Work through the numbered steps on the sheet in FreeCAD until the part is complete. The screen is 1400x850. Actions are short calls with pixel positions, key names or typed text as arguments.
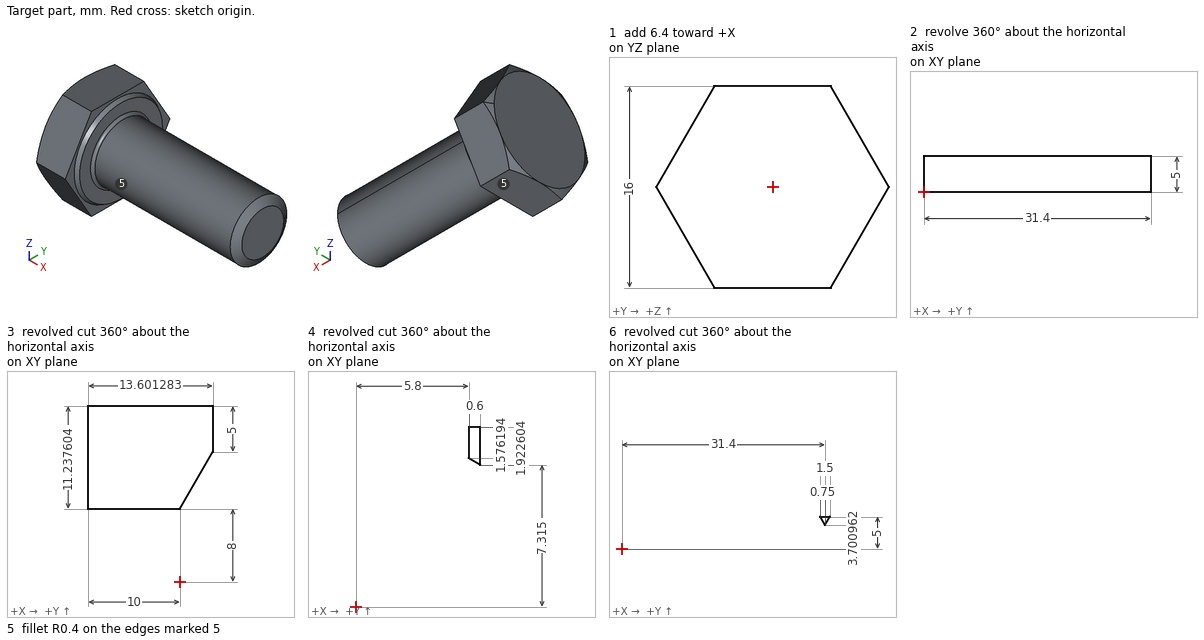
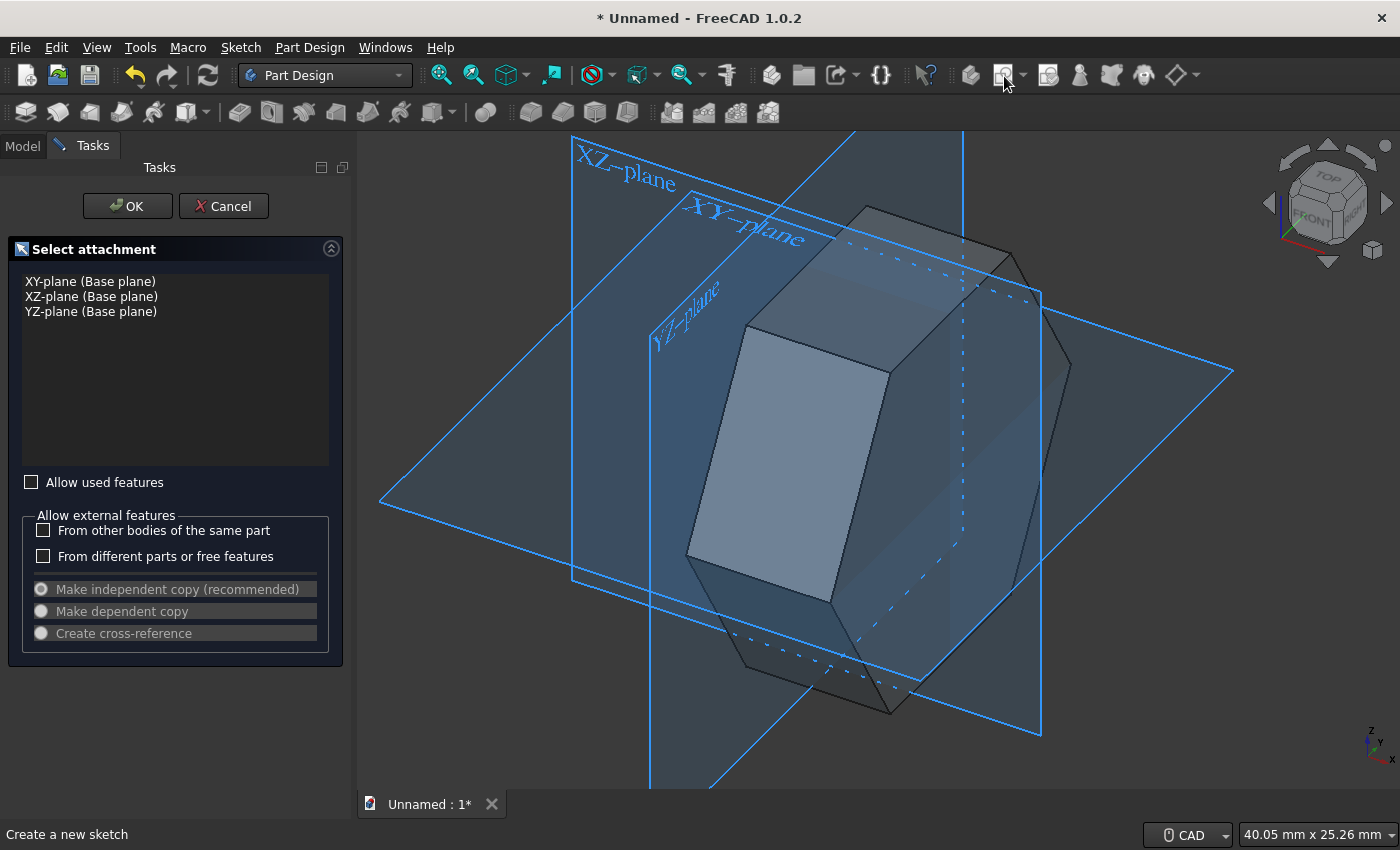
click(82, 282)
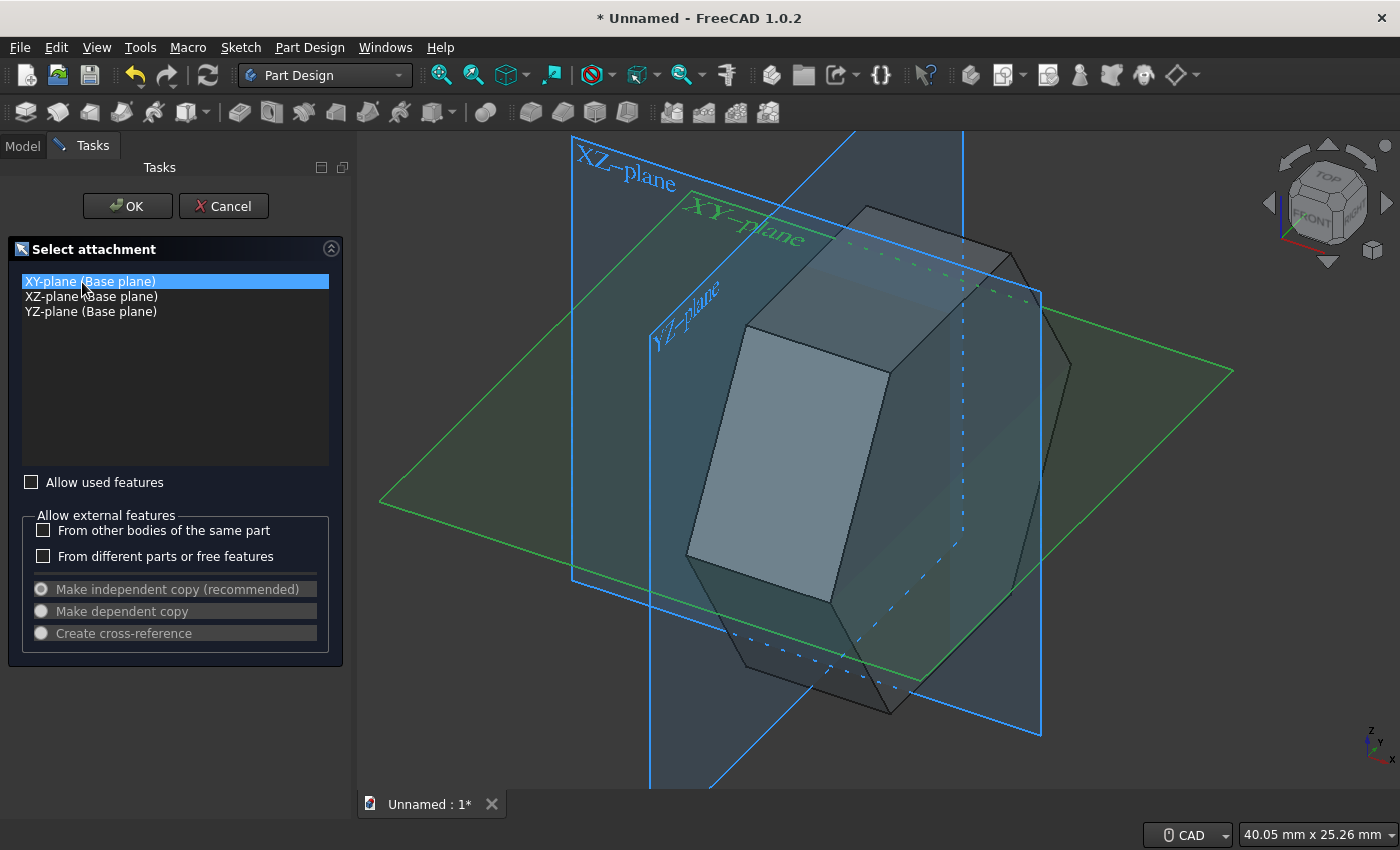
click(128, 206)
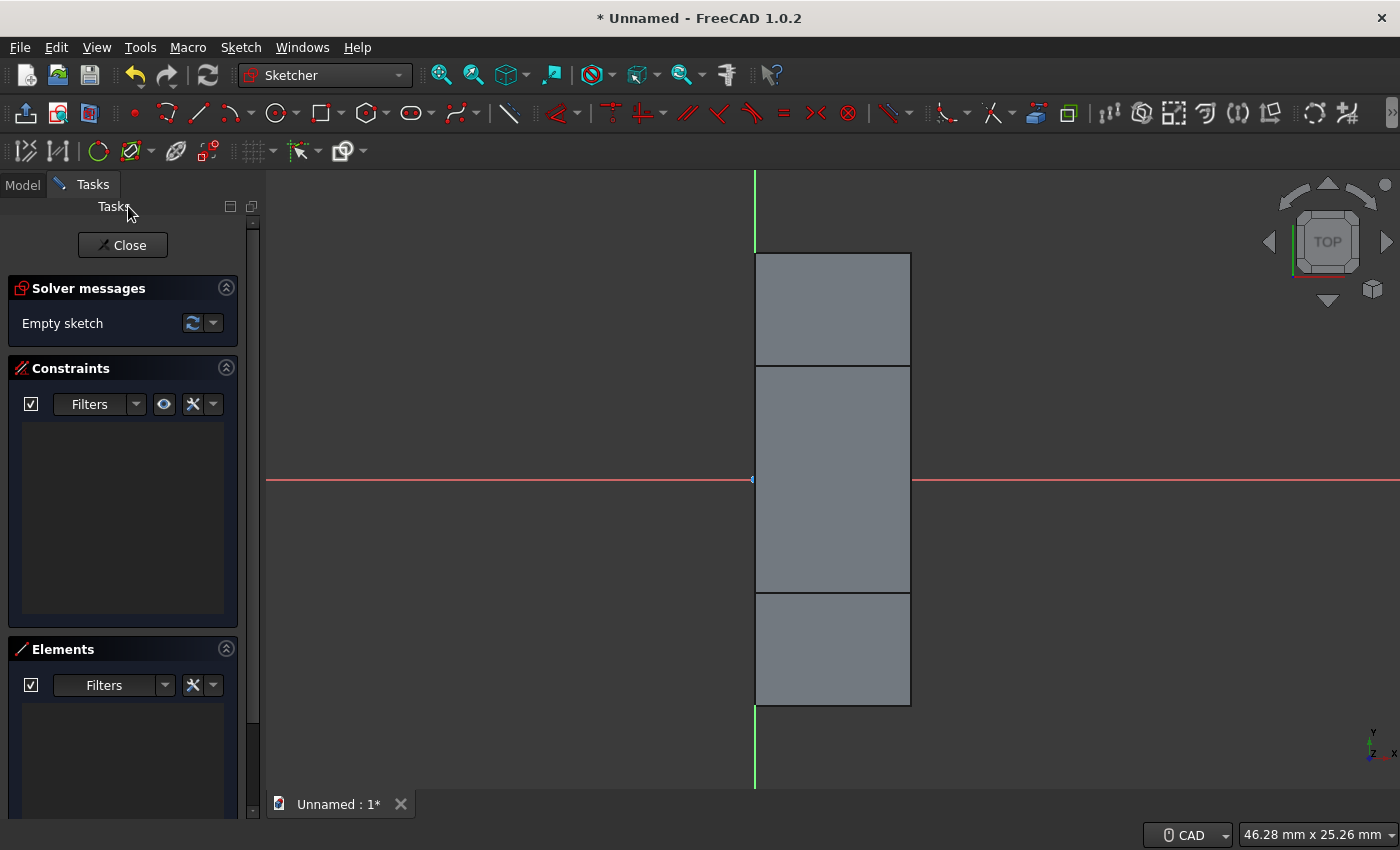
click(90, 114)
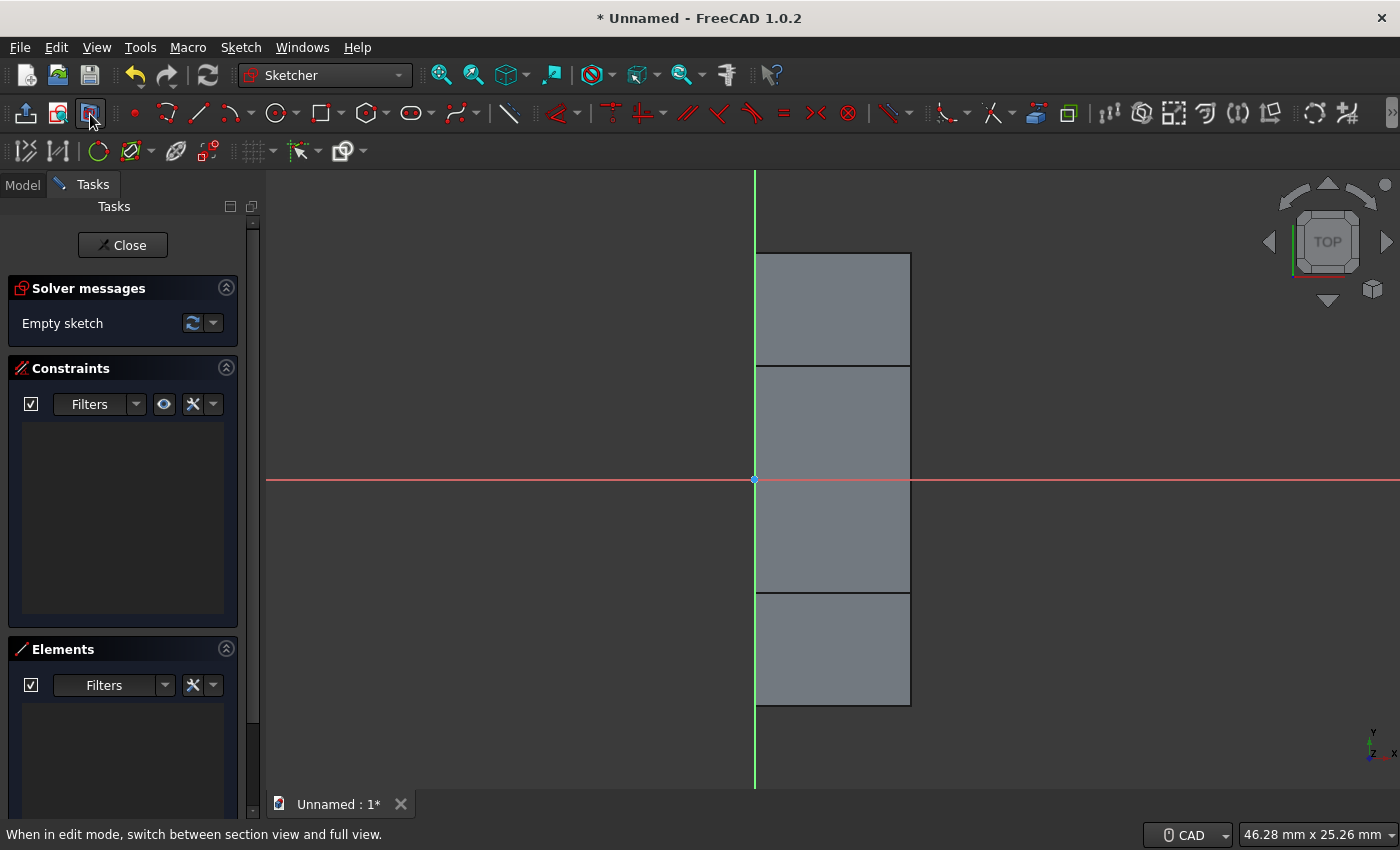
scroll(294, 604, down, 2)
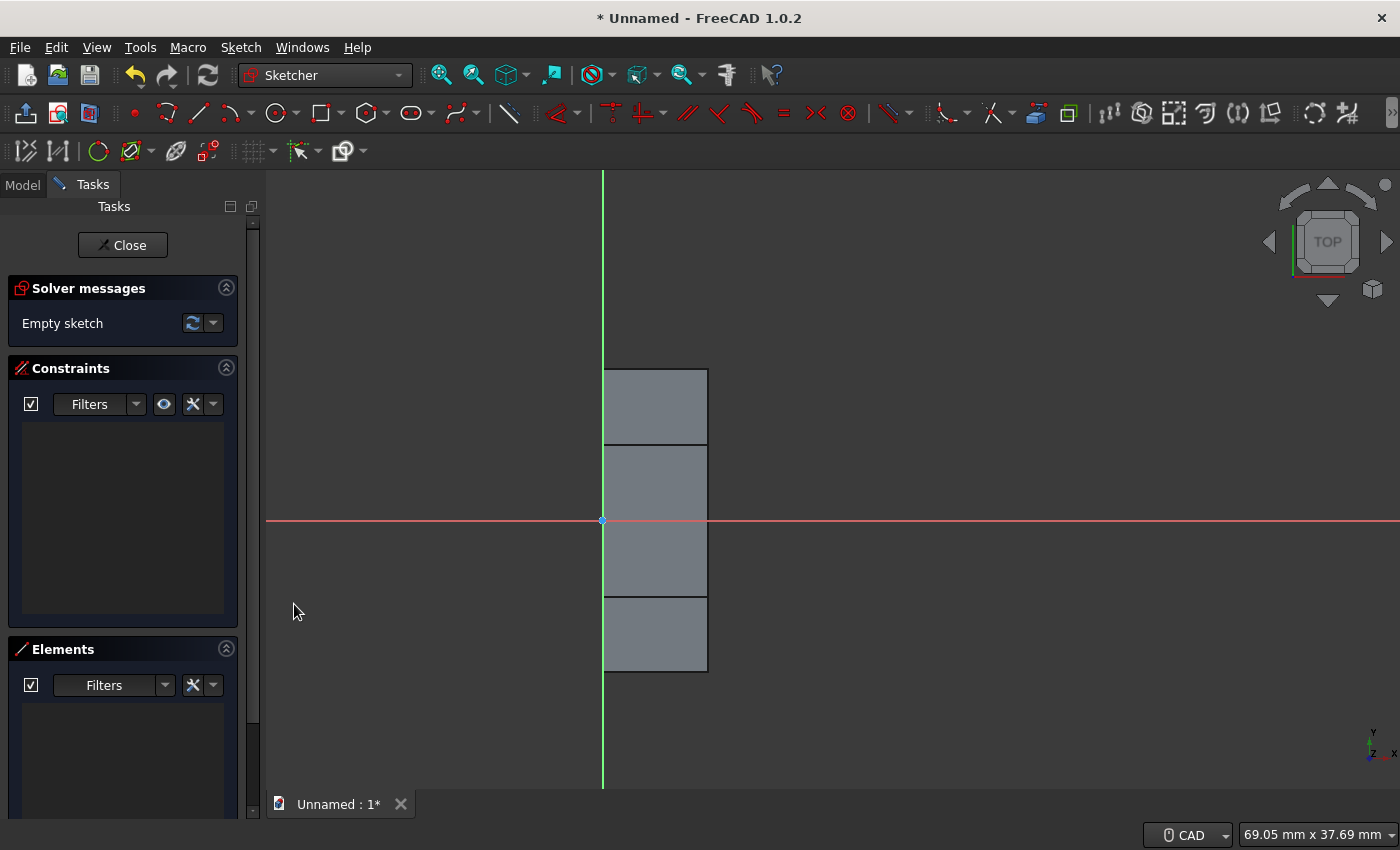
click(322, 114)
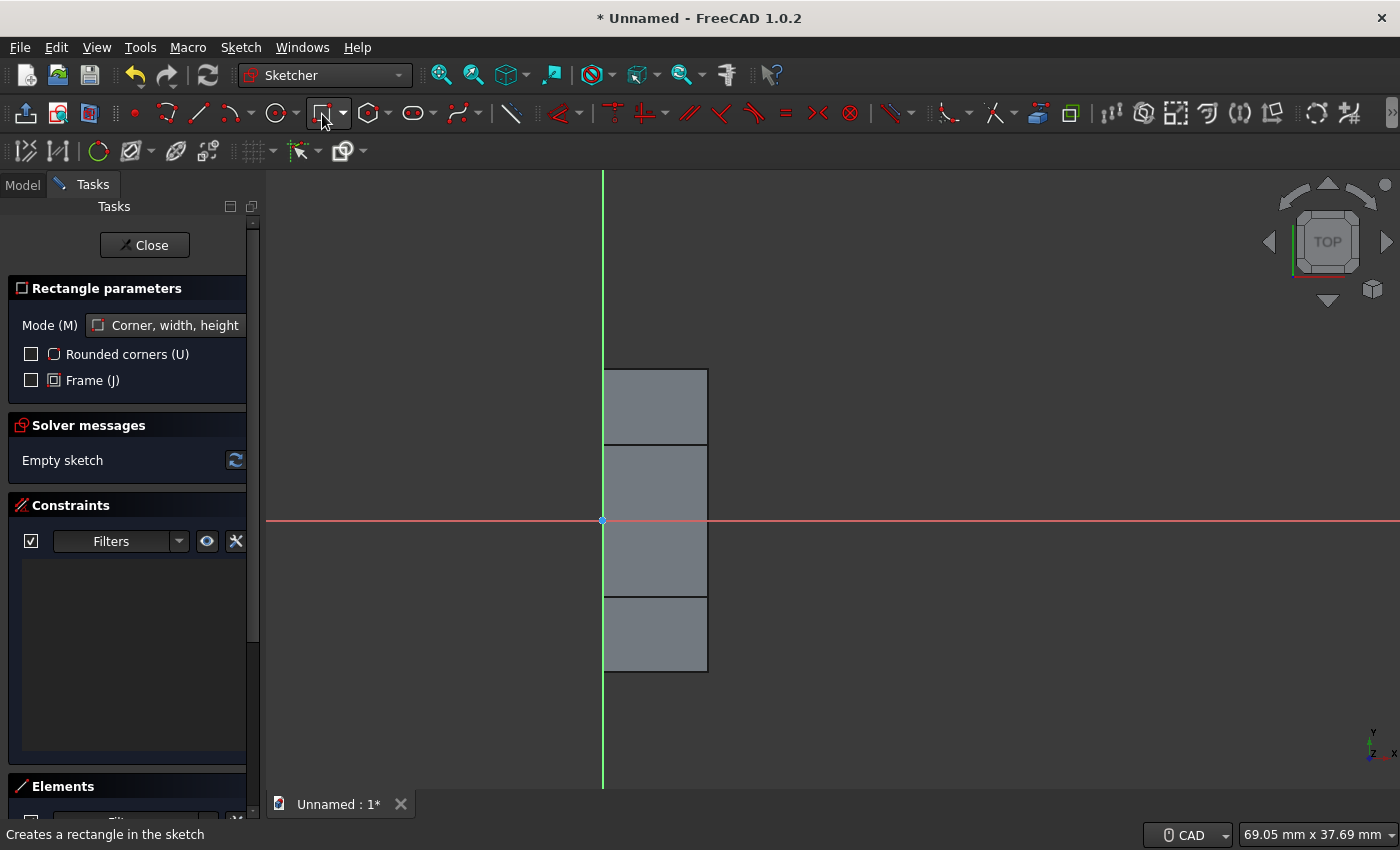
click(603, 521)
click(1118, 439)
key(Escape)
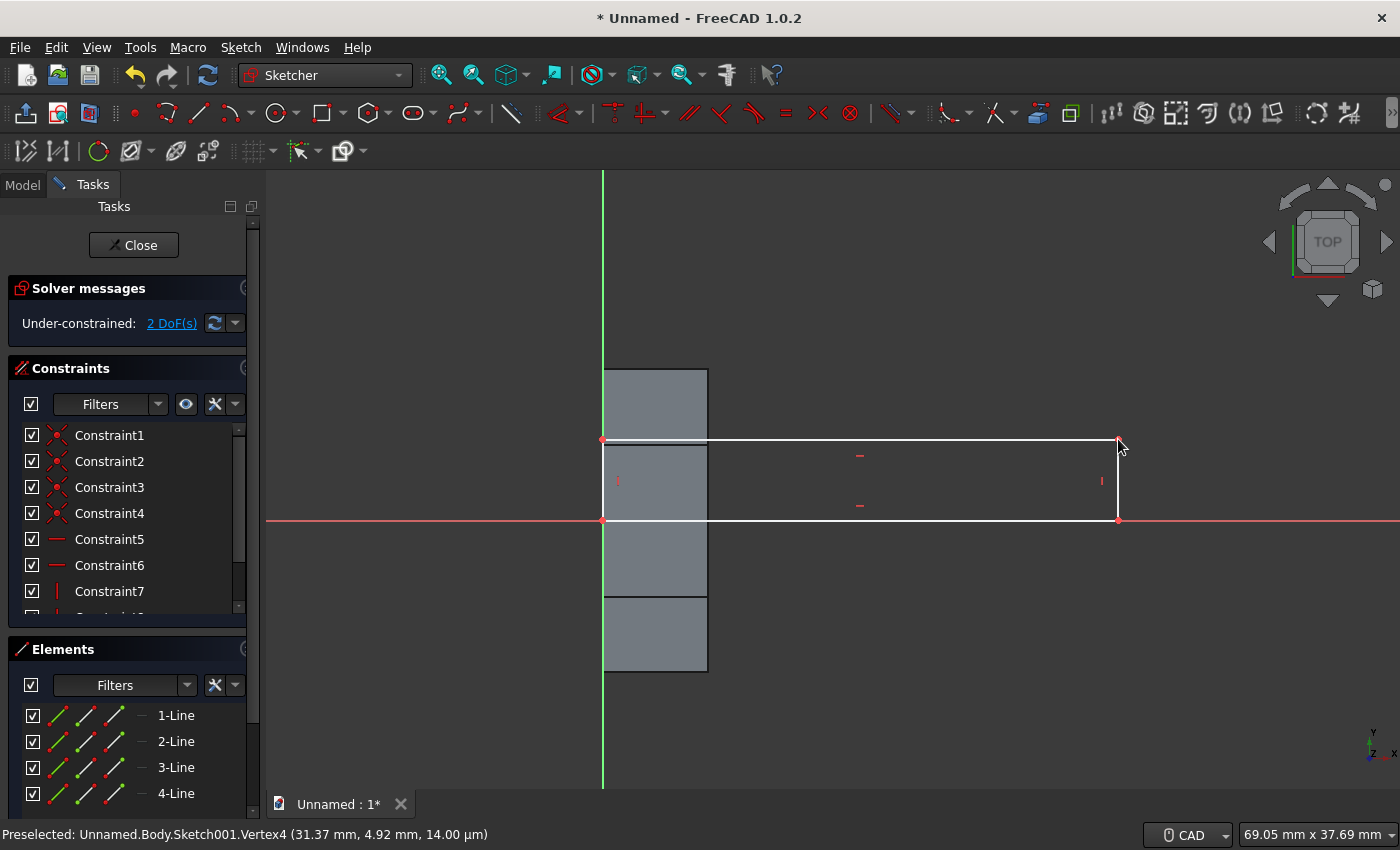
click(558, 114)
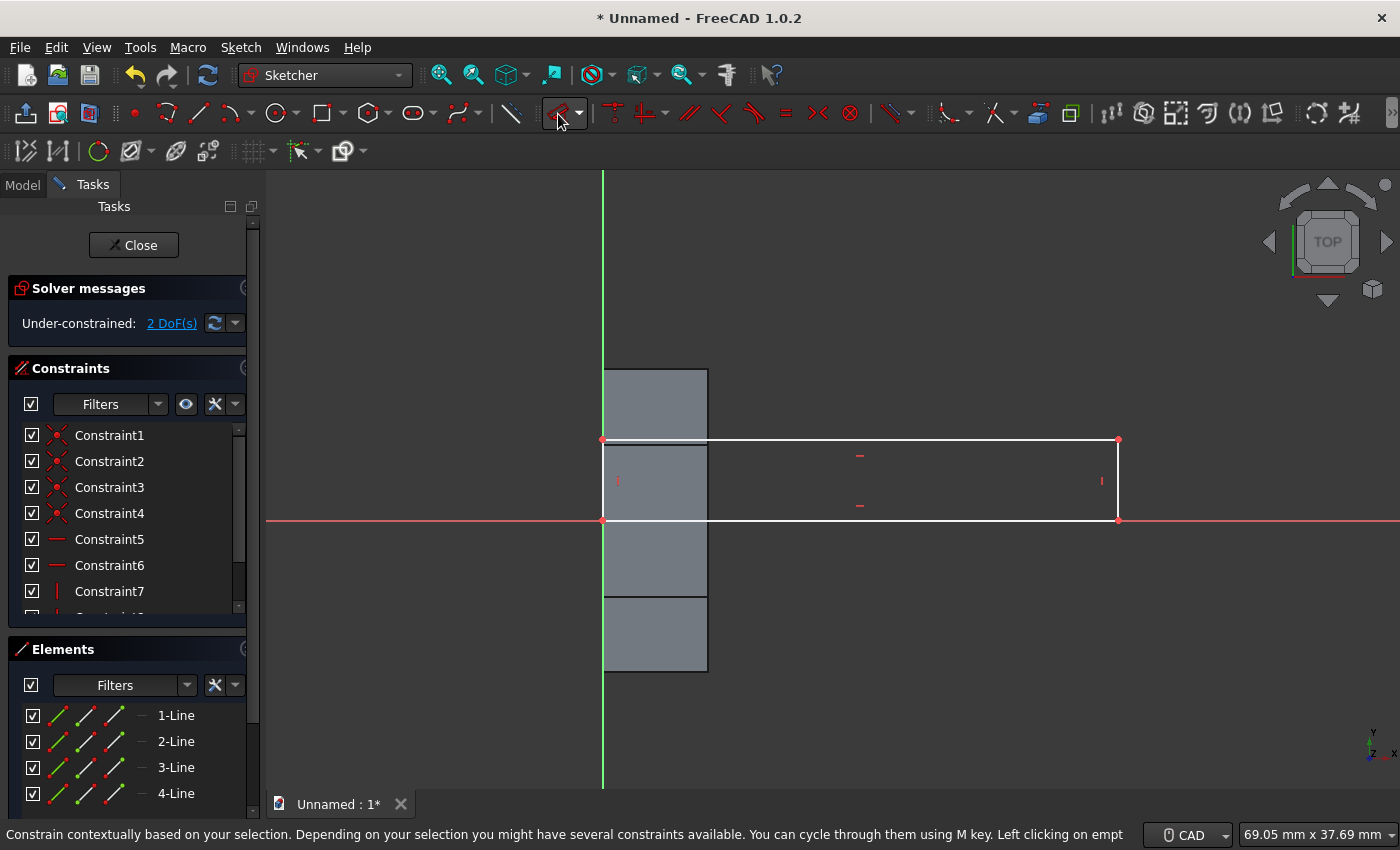
click(1118, 497)
click(1152, 480)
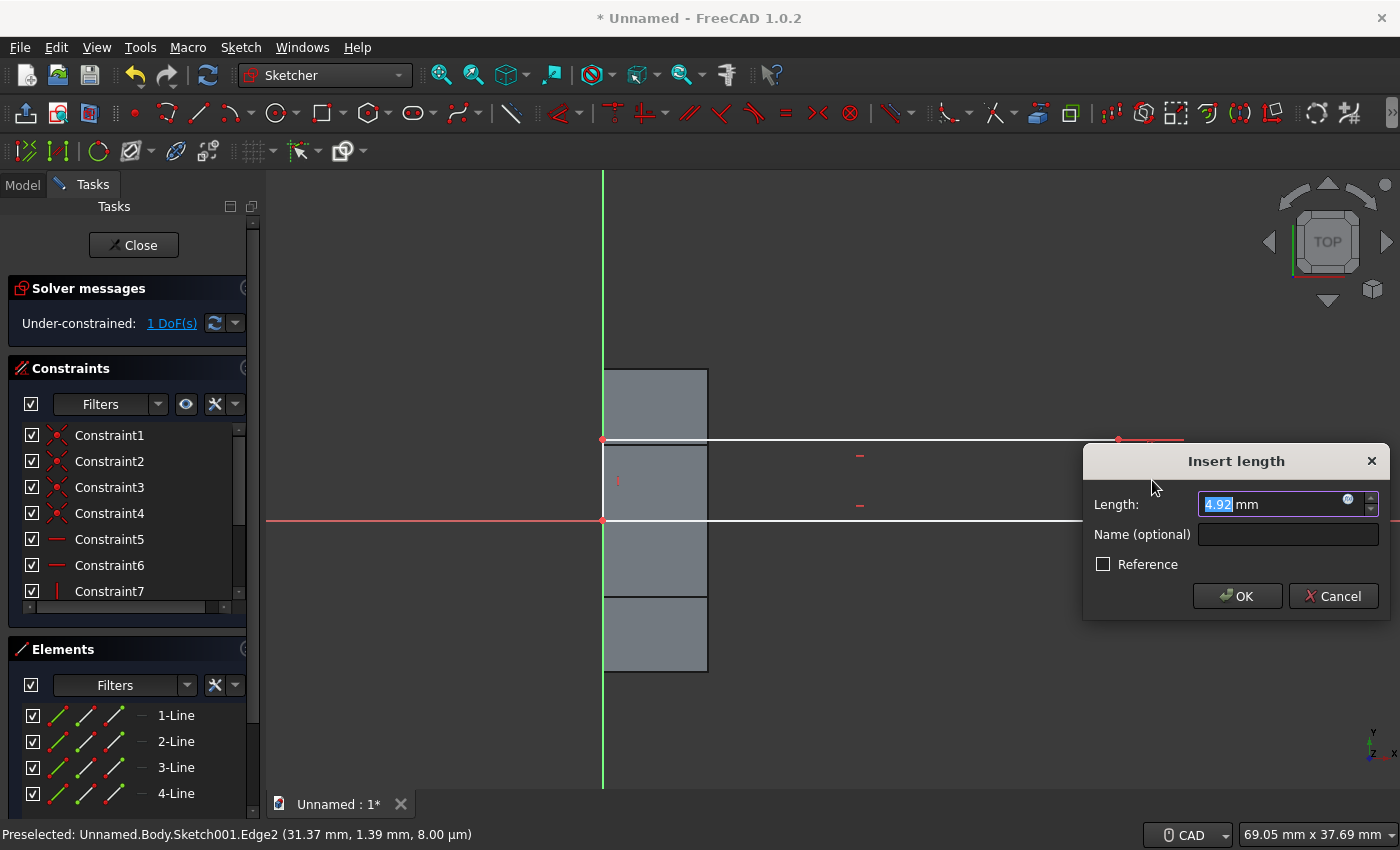
text(5)
key(Return)